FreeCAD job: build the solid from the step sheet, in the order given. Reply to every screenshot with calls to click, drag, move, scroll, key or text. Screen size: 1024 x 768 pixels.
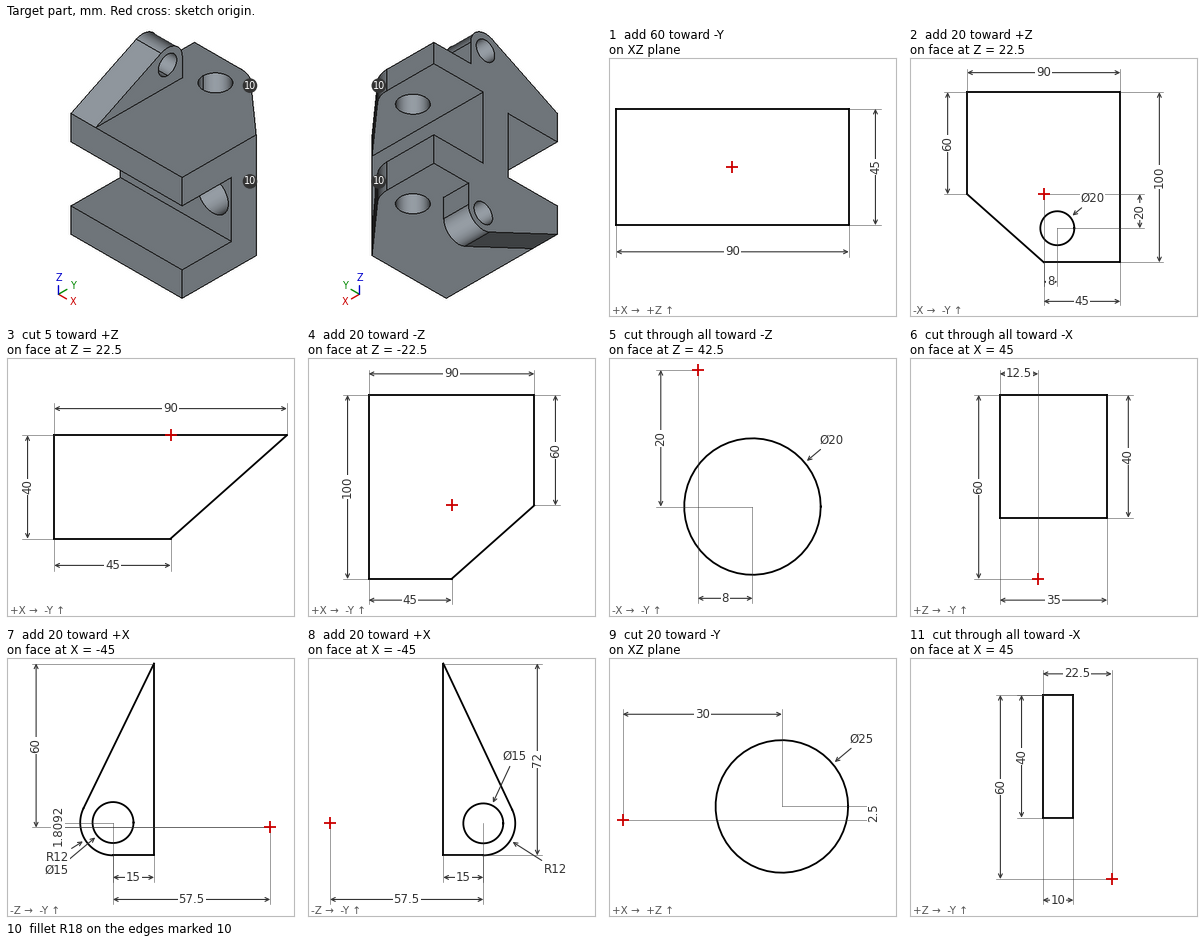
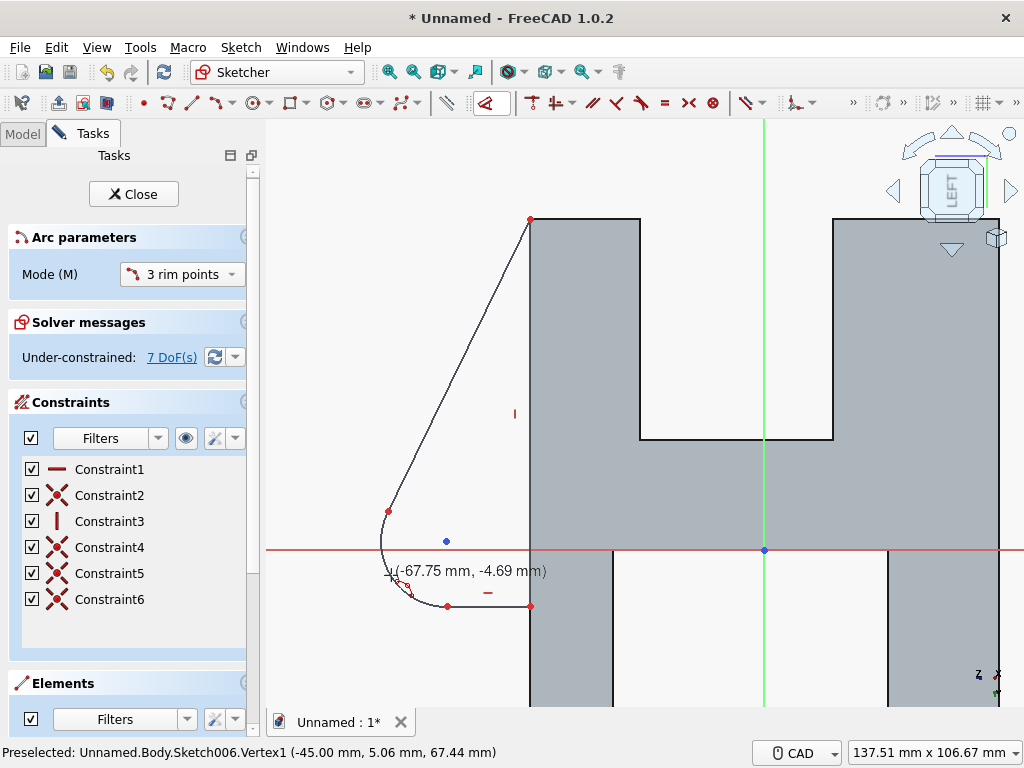
click(254, 104)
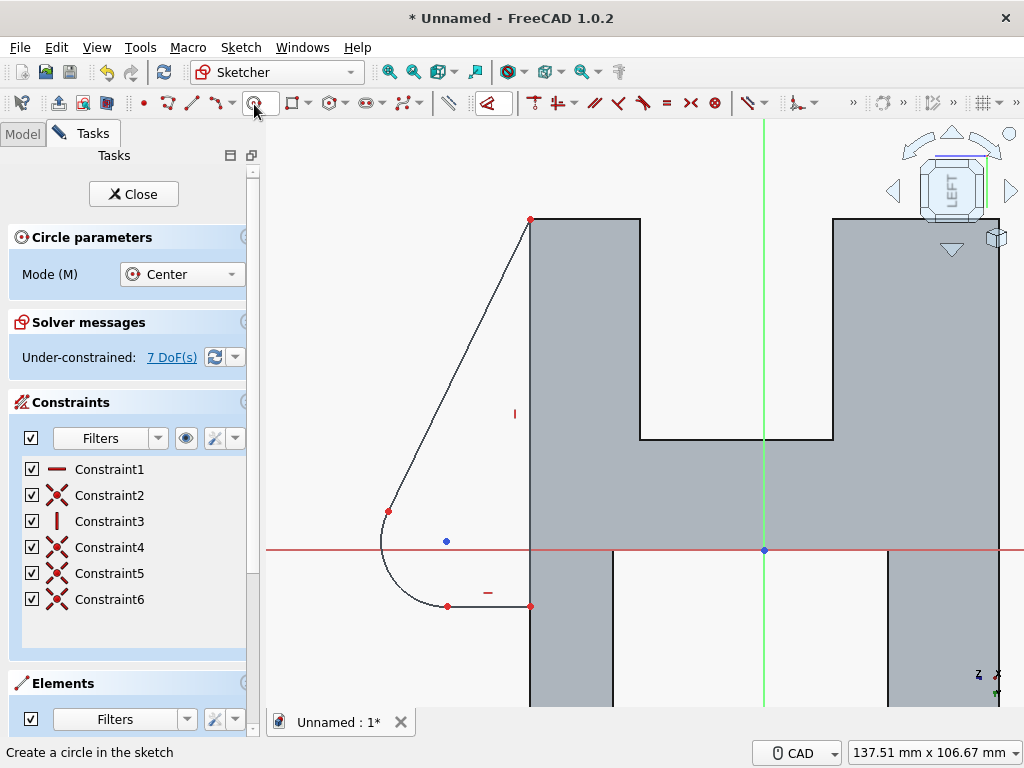
scroll(447, 540, up, 3)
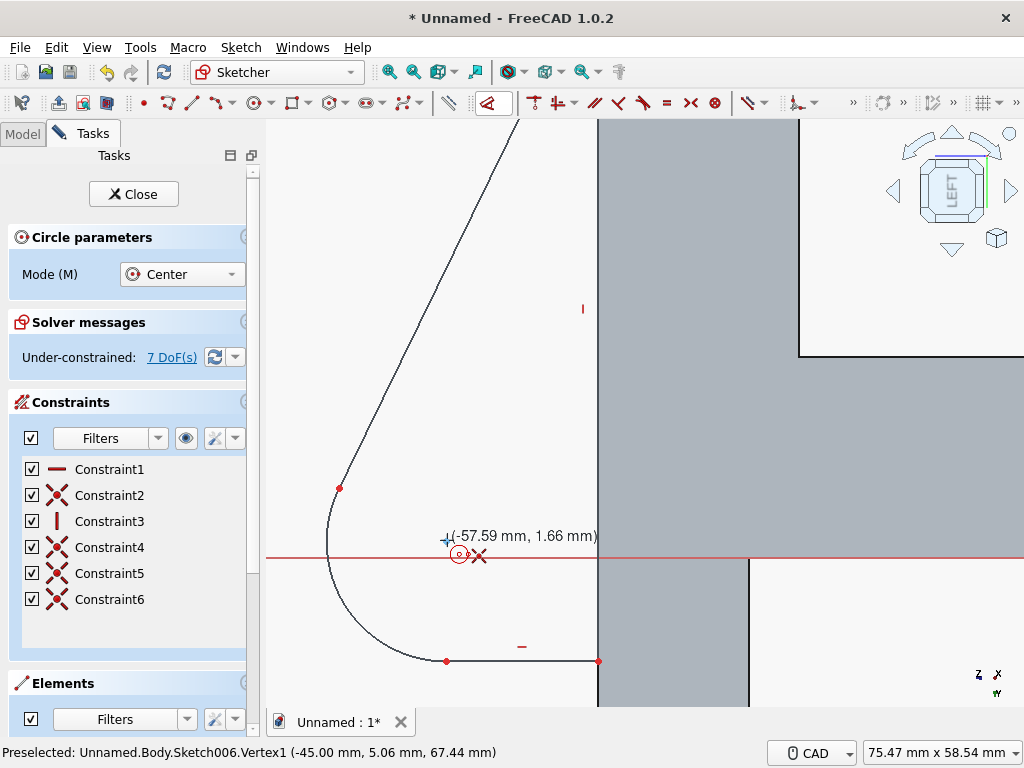
click(448, 540)
move(501, 486)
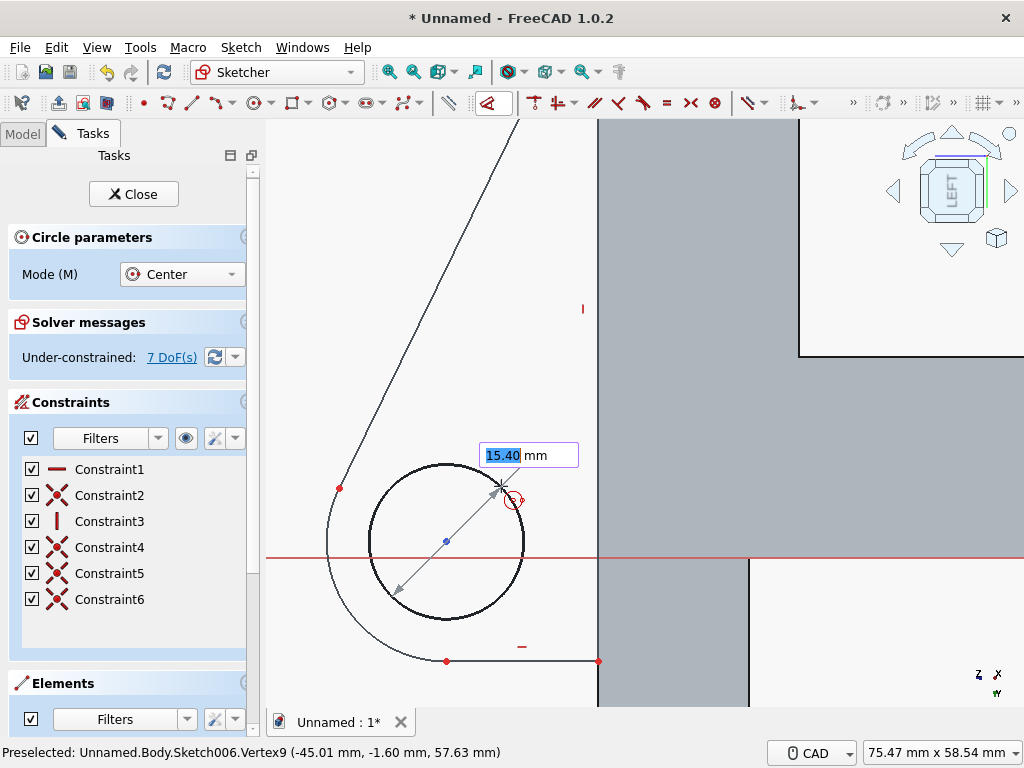
text(15)
key(Return)
key(Escape)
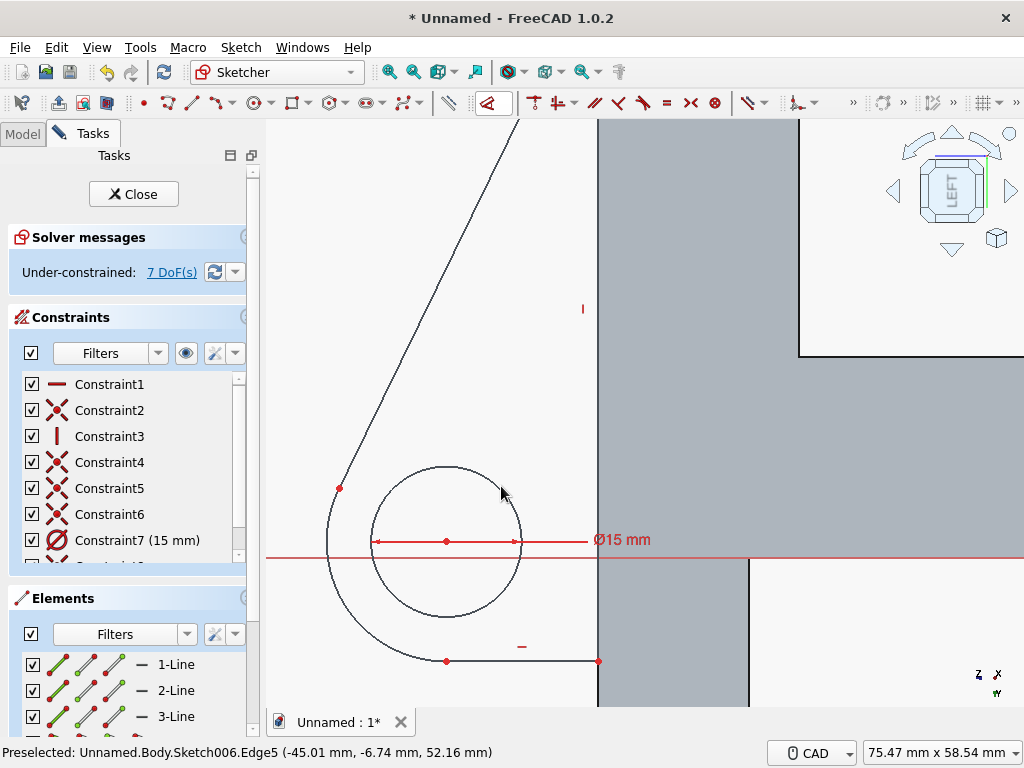
click(492, 661)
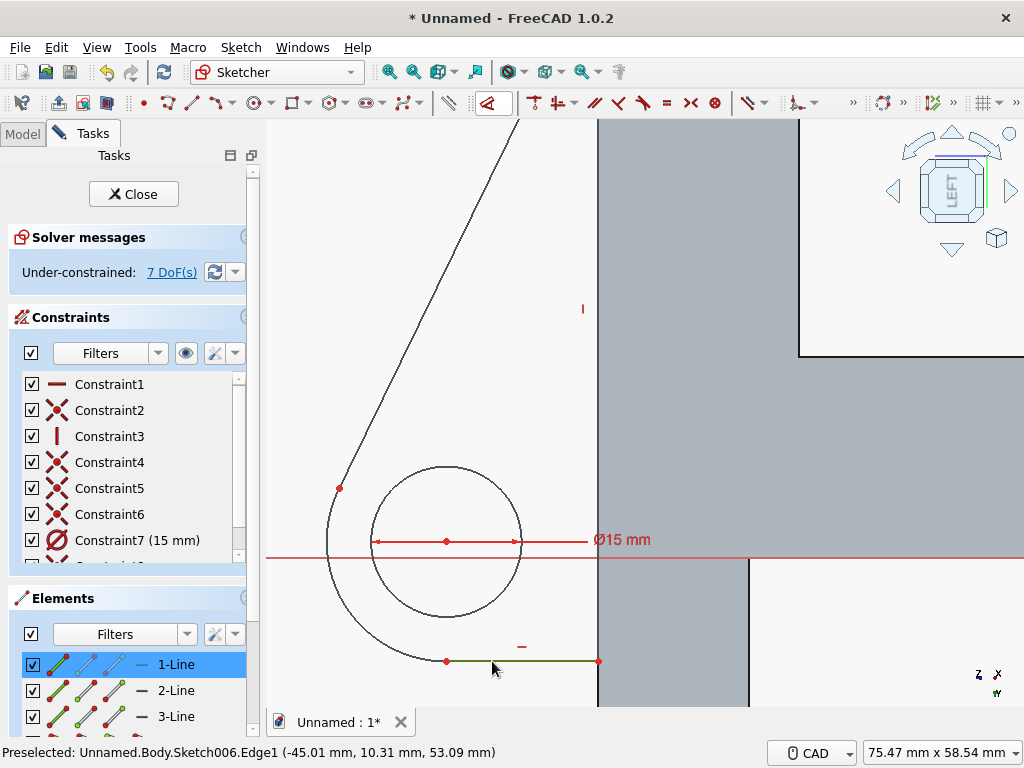
click(328, 560)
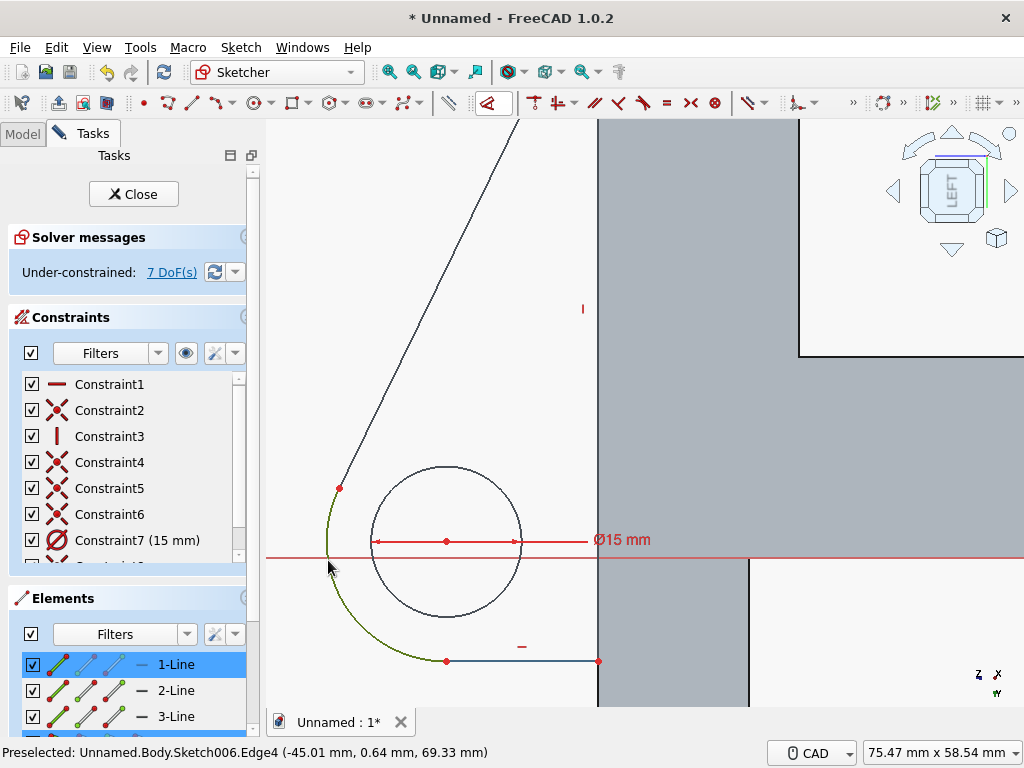
key(t)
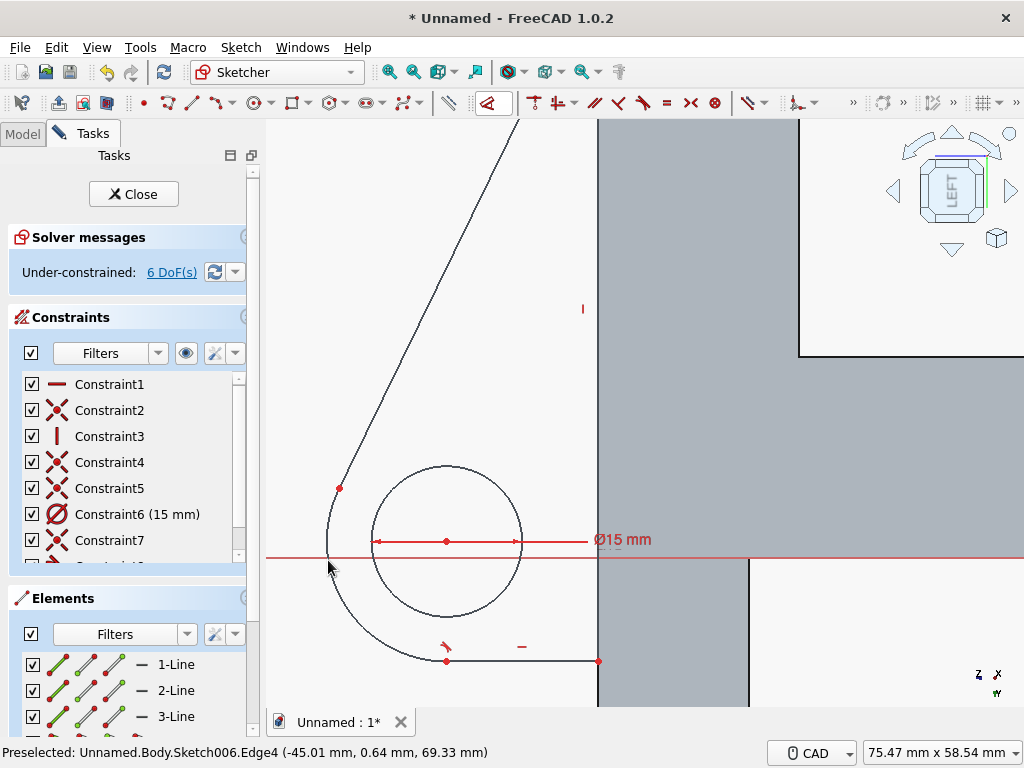
click(417, 329)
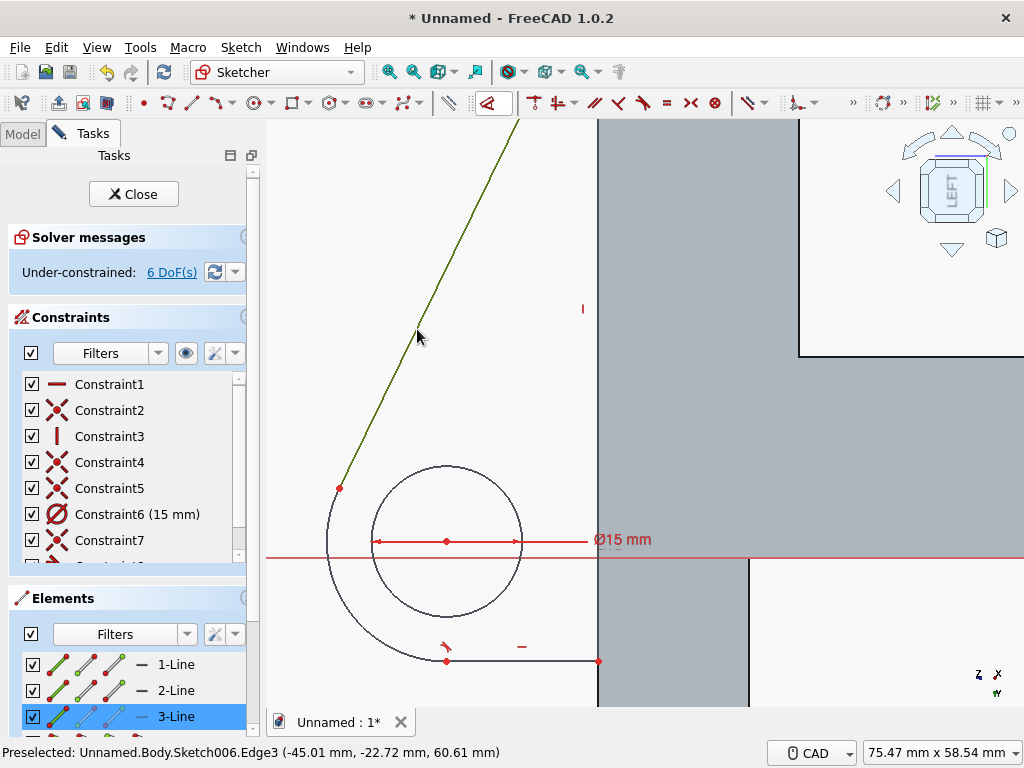
click(328, 559)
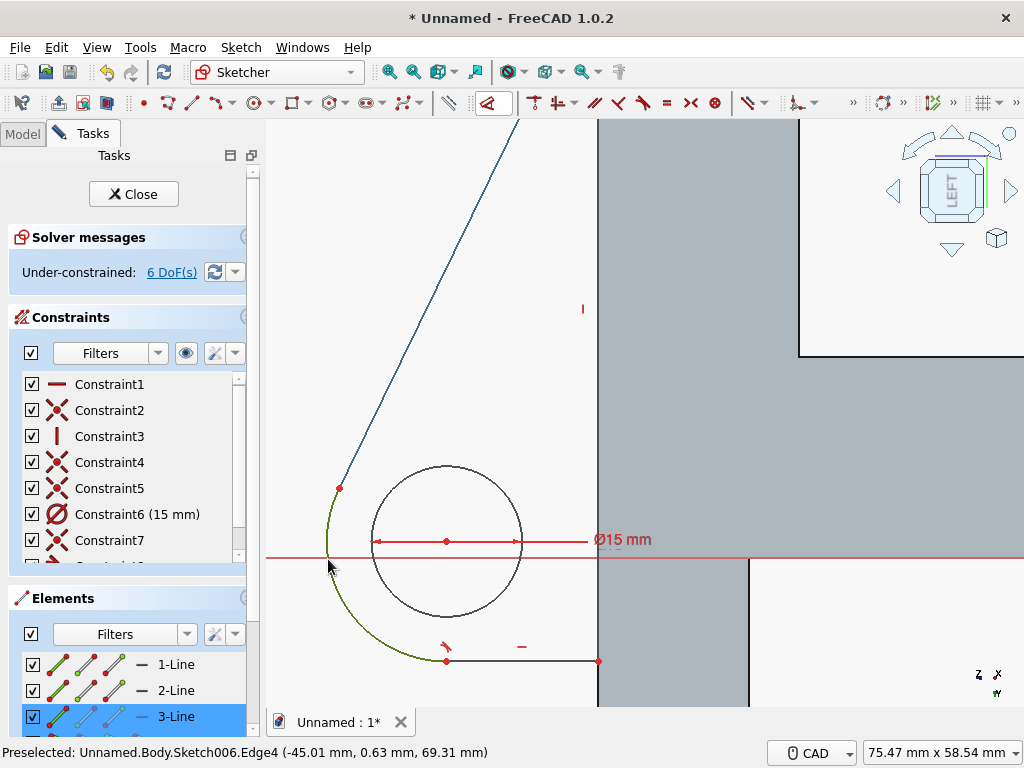
key(t)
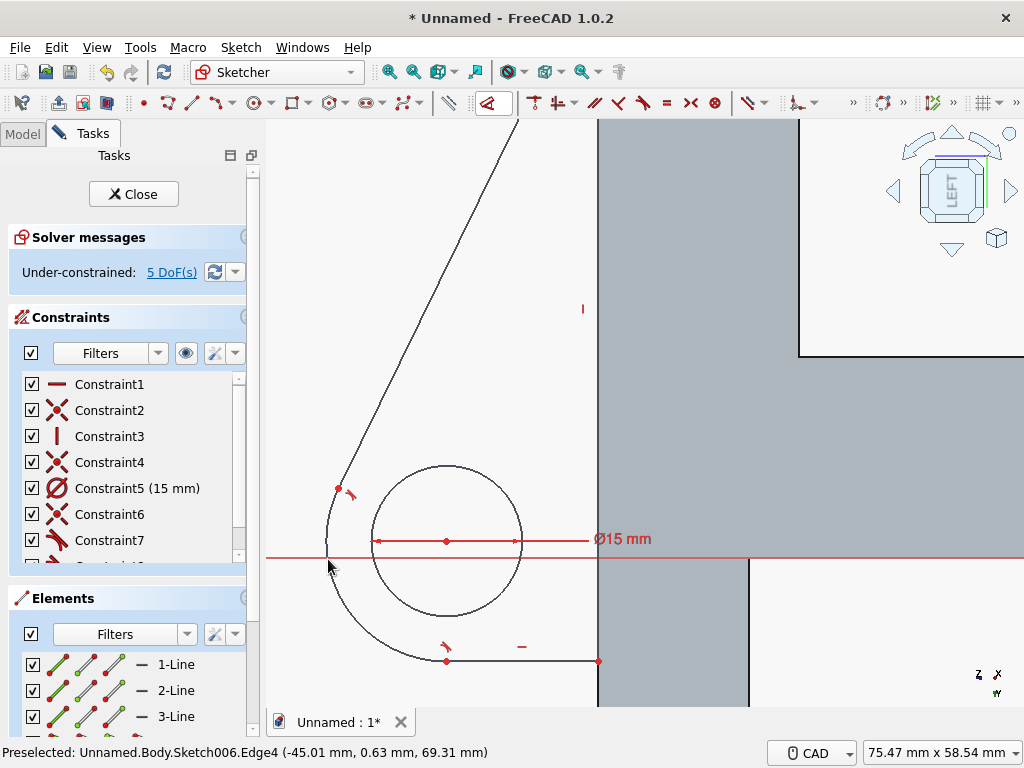
click(328, 560)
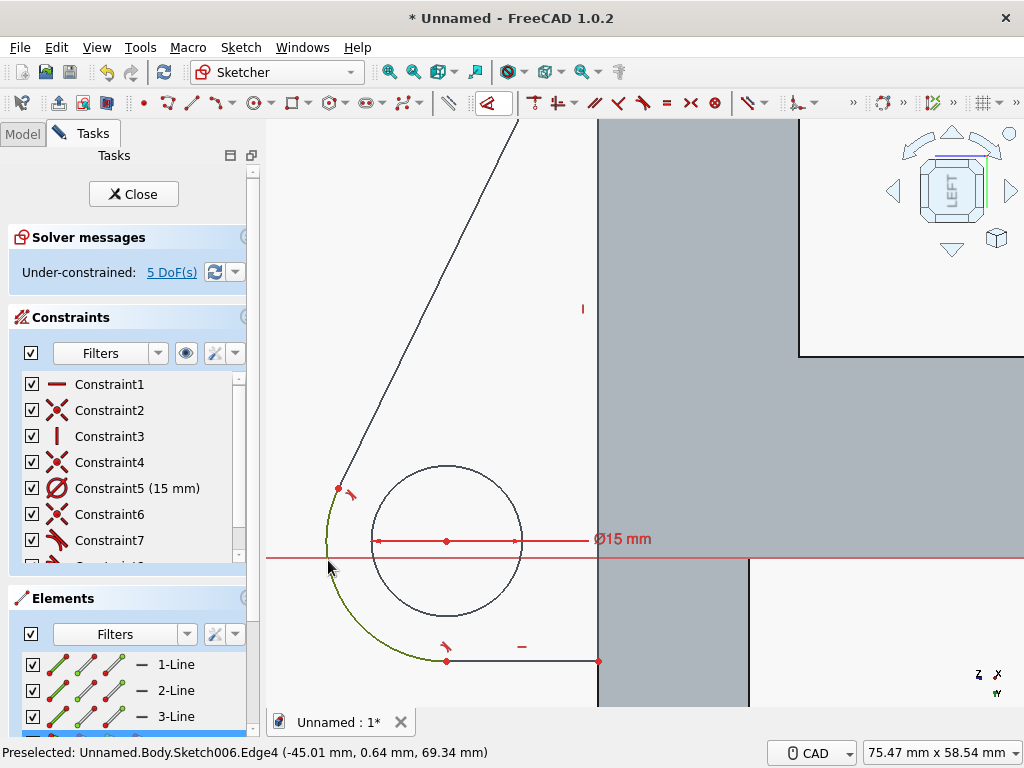
click(506, 104)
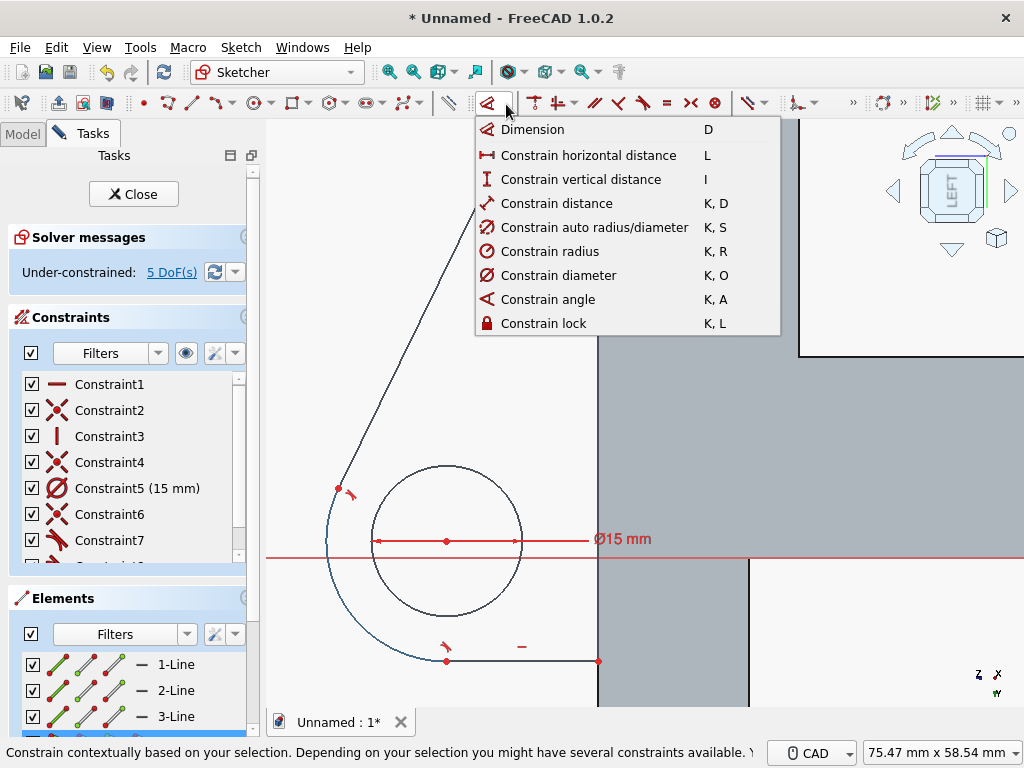
click(628, 251)